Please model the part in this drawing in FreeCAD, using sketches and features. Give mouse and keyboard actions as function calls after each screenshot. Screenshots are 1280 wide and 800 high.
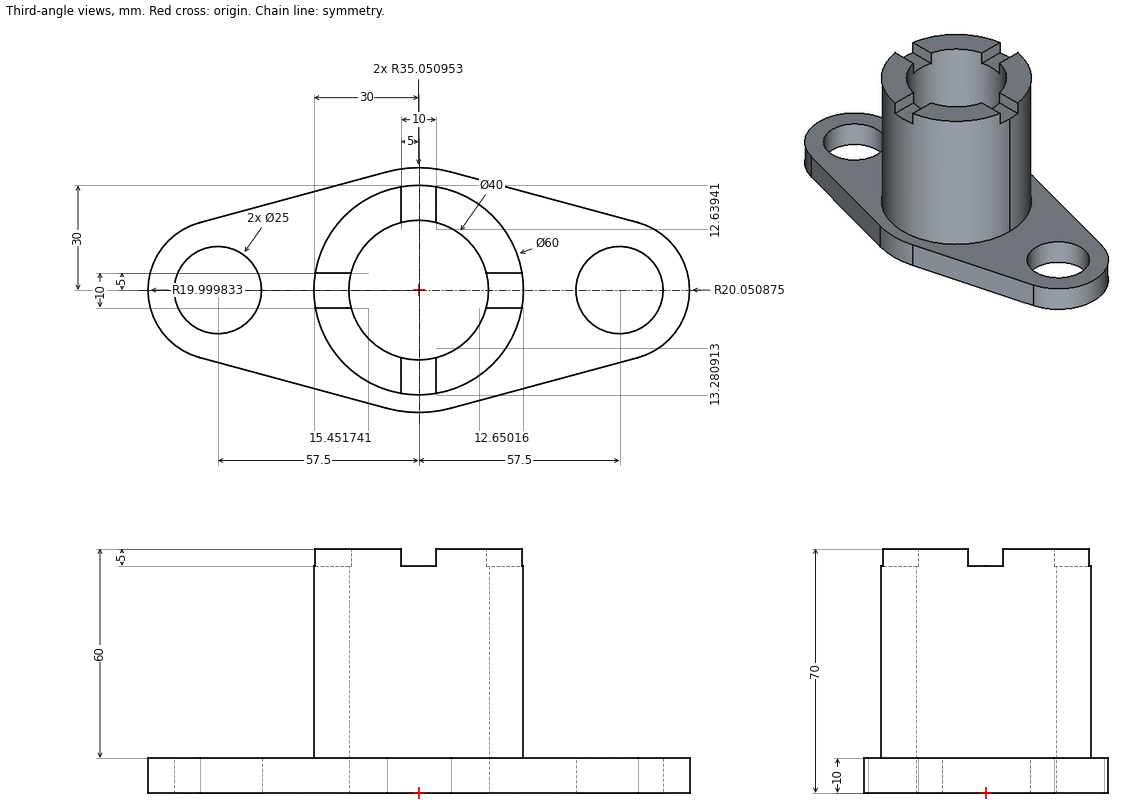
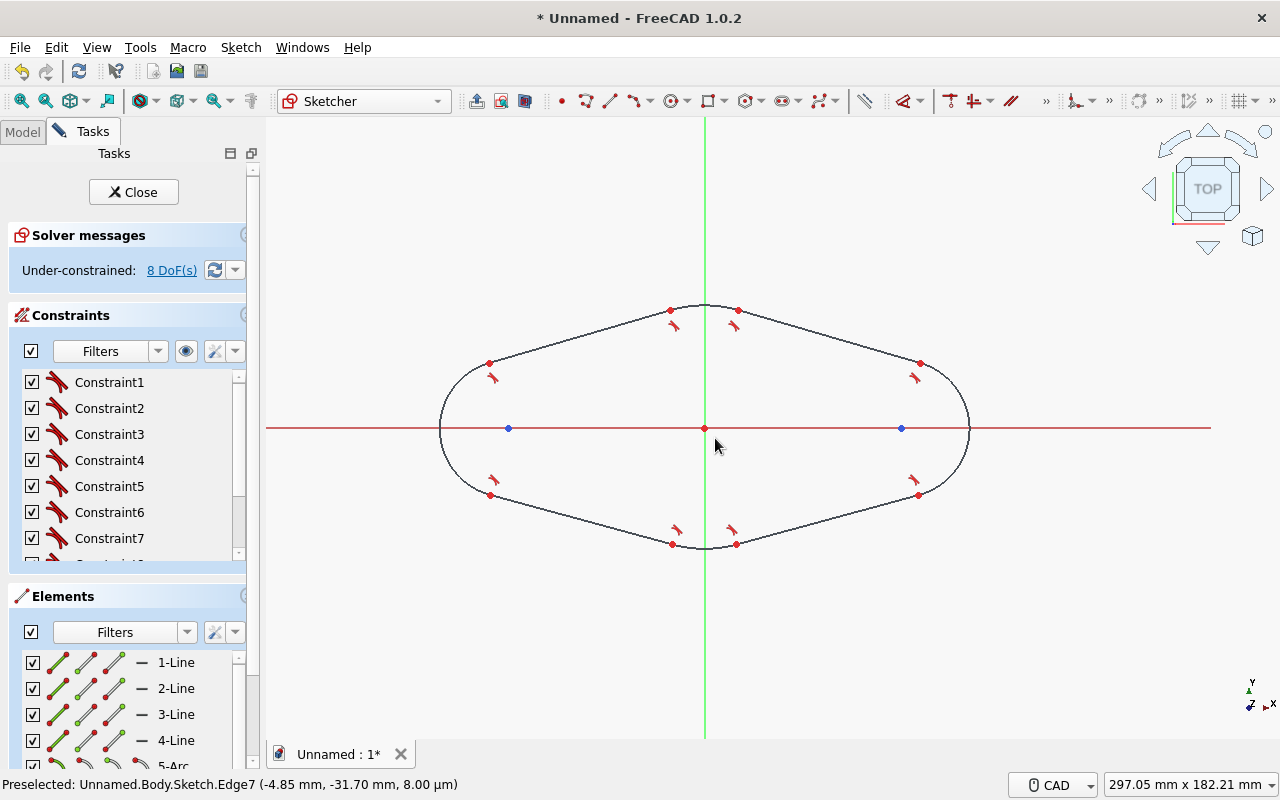
click(718, 306)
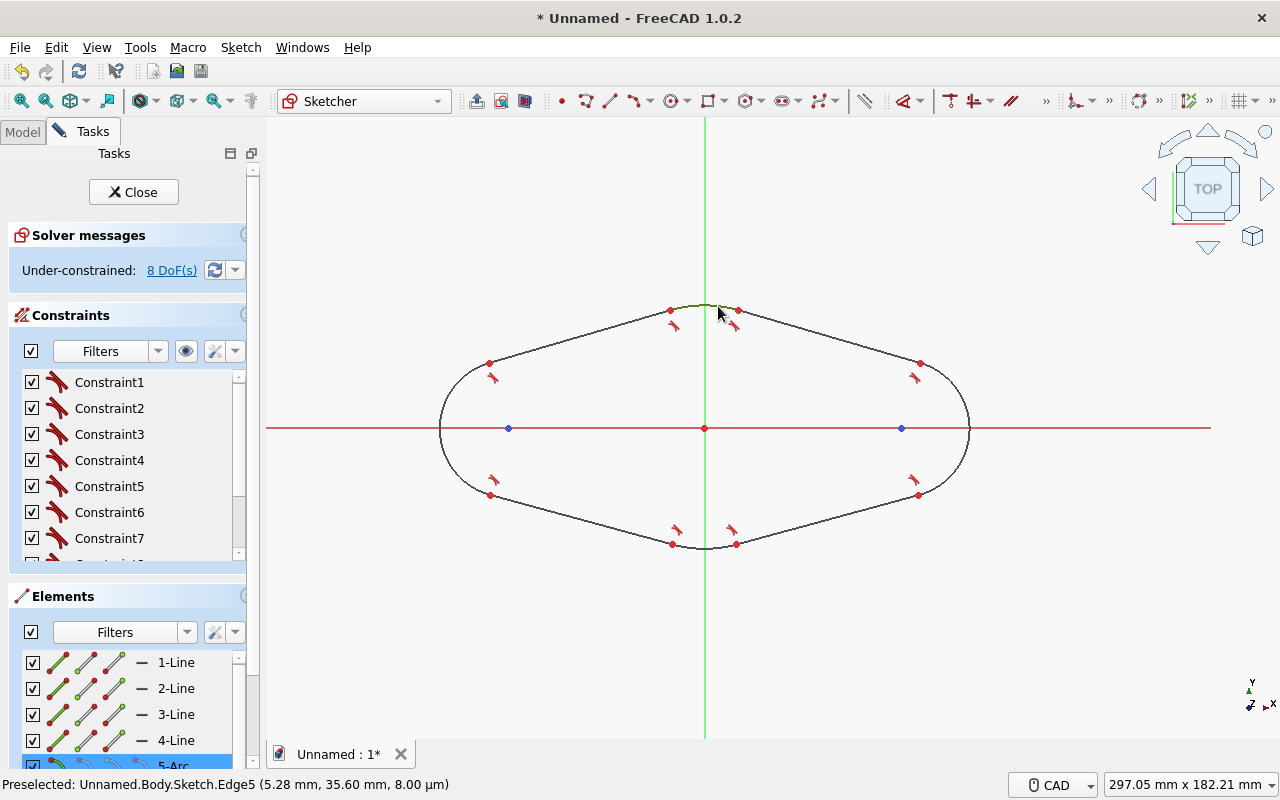
click(692, 548)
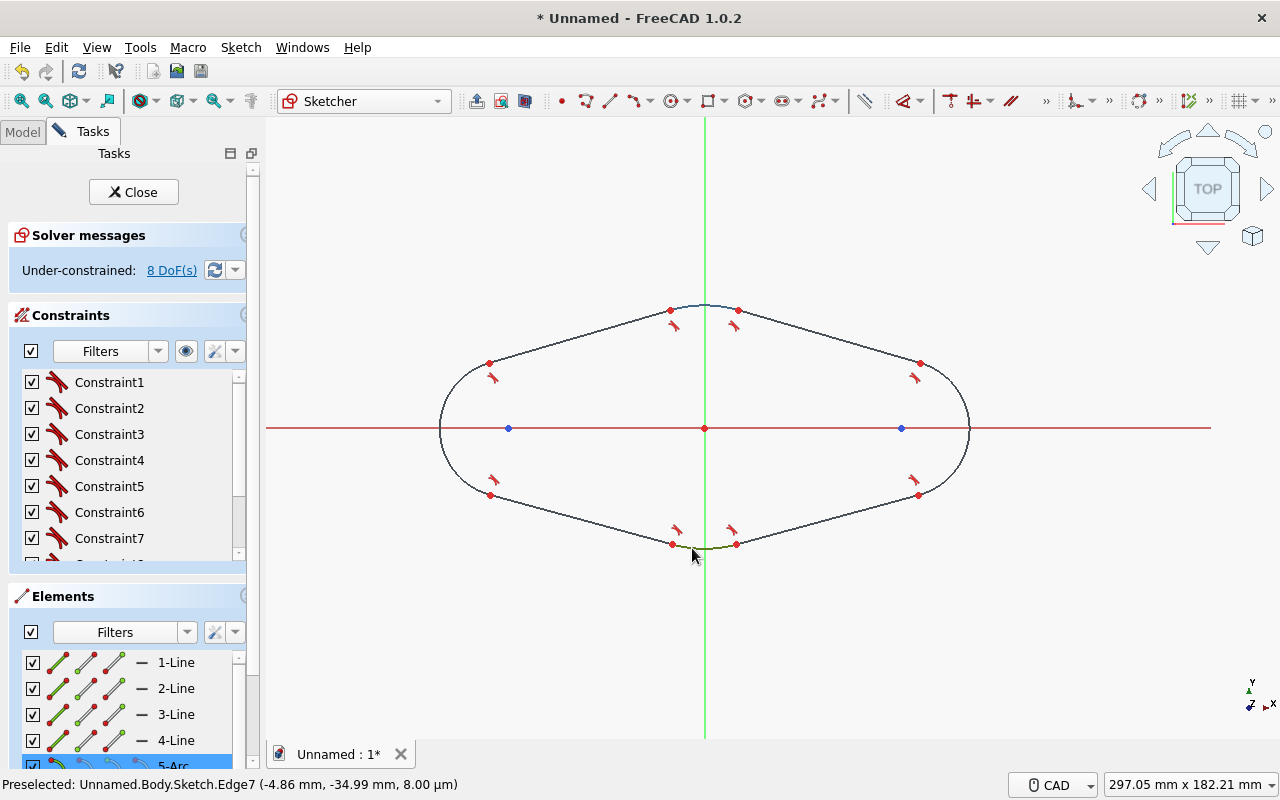
key(e)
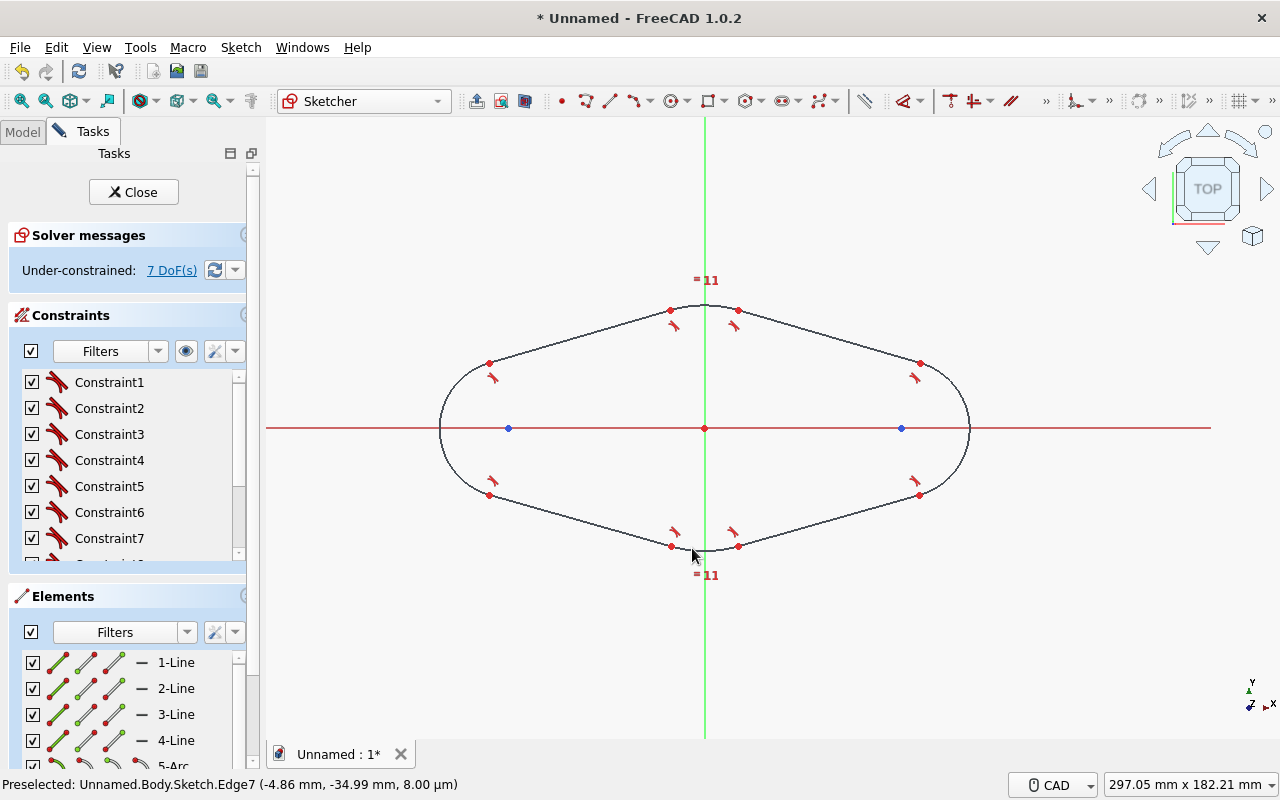
click(508, 429)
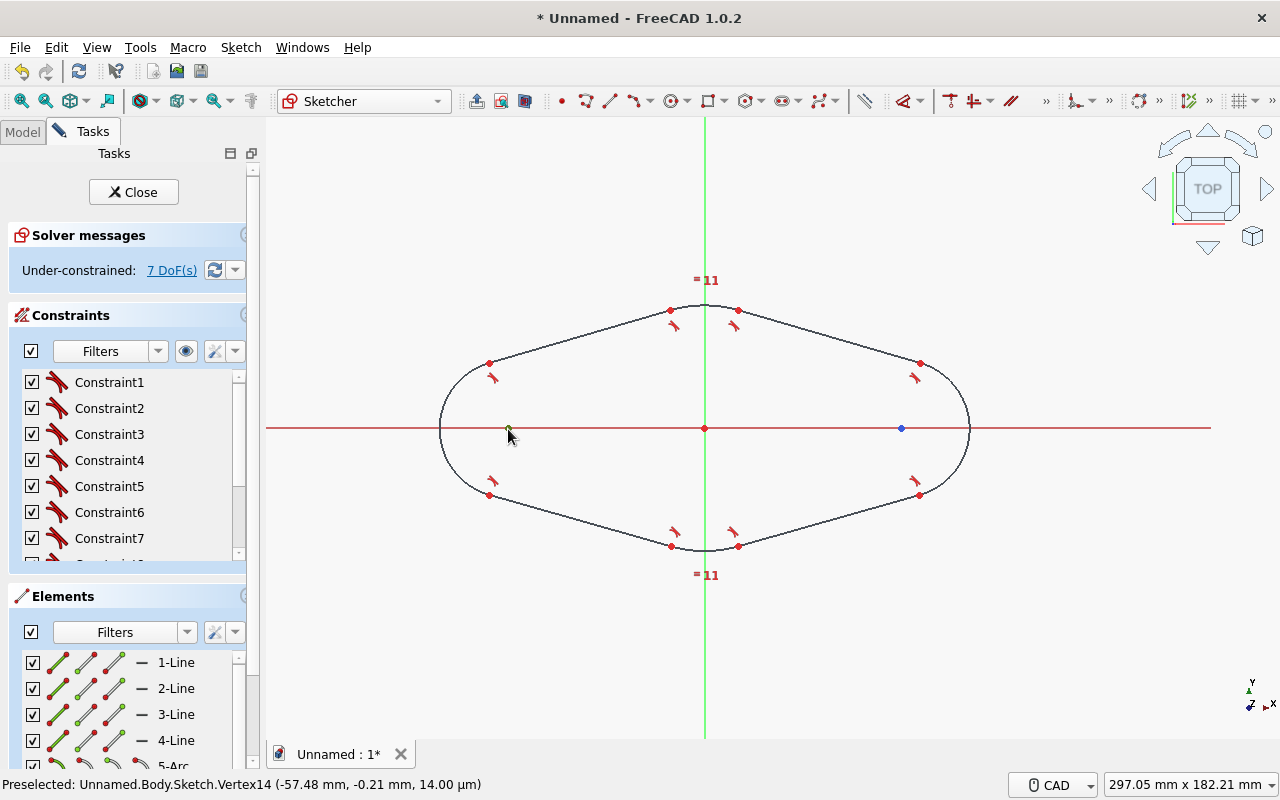
click(353, 428)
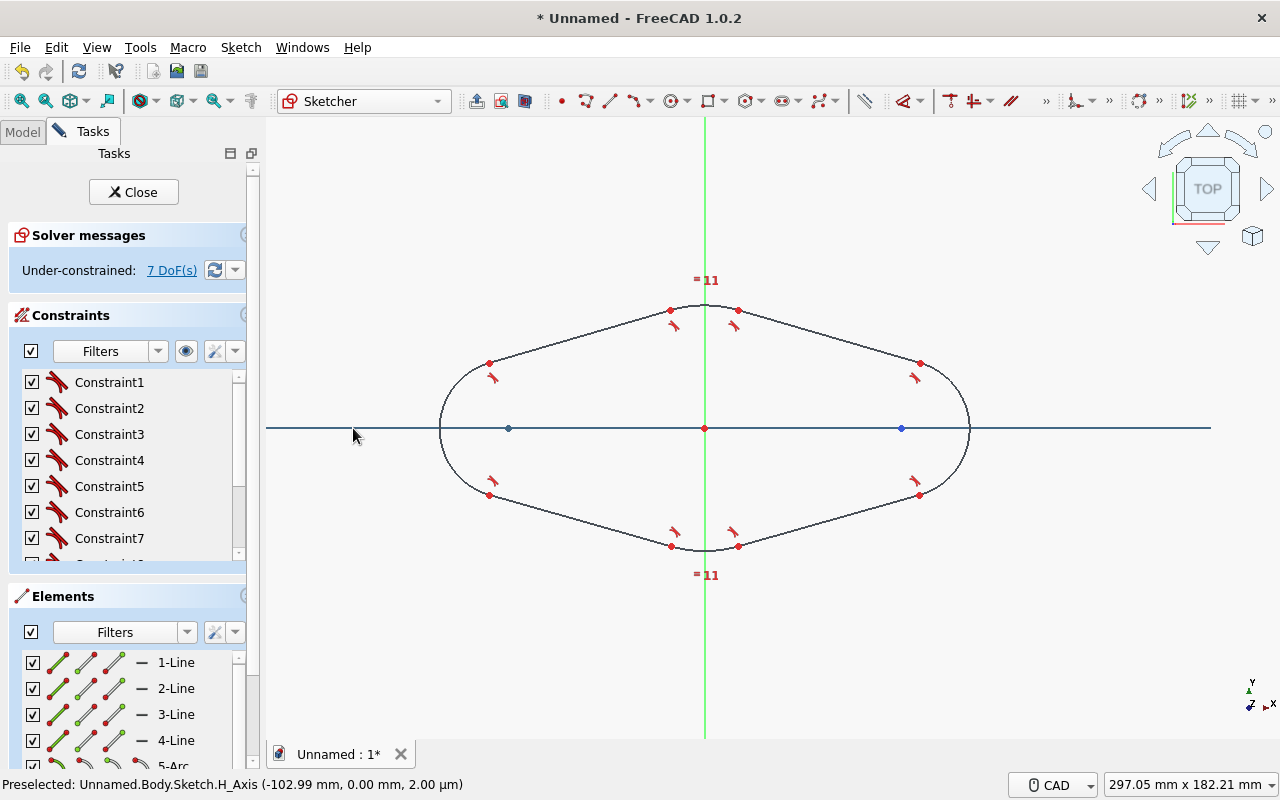
key(c)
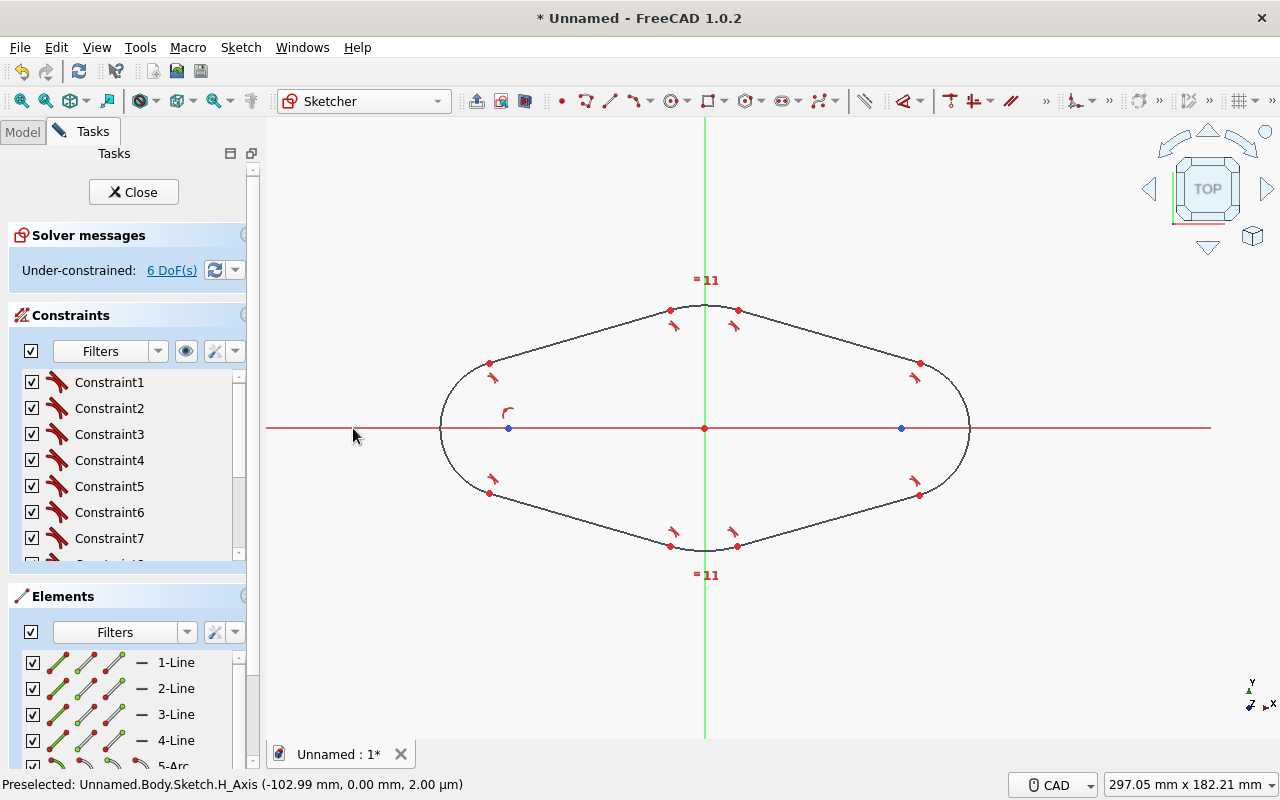
click(901, 429)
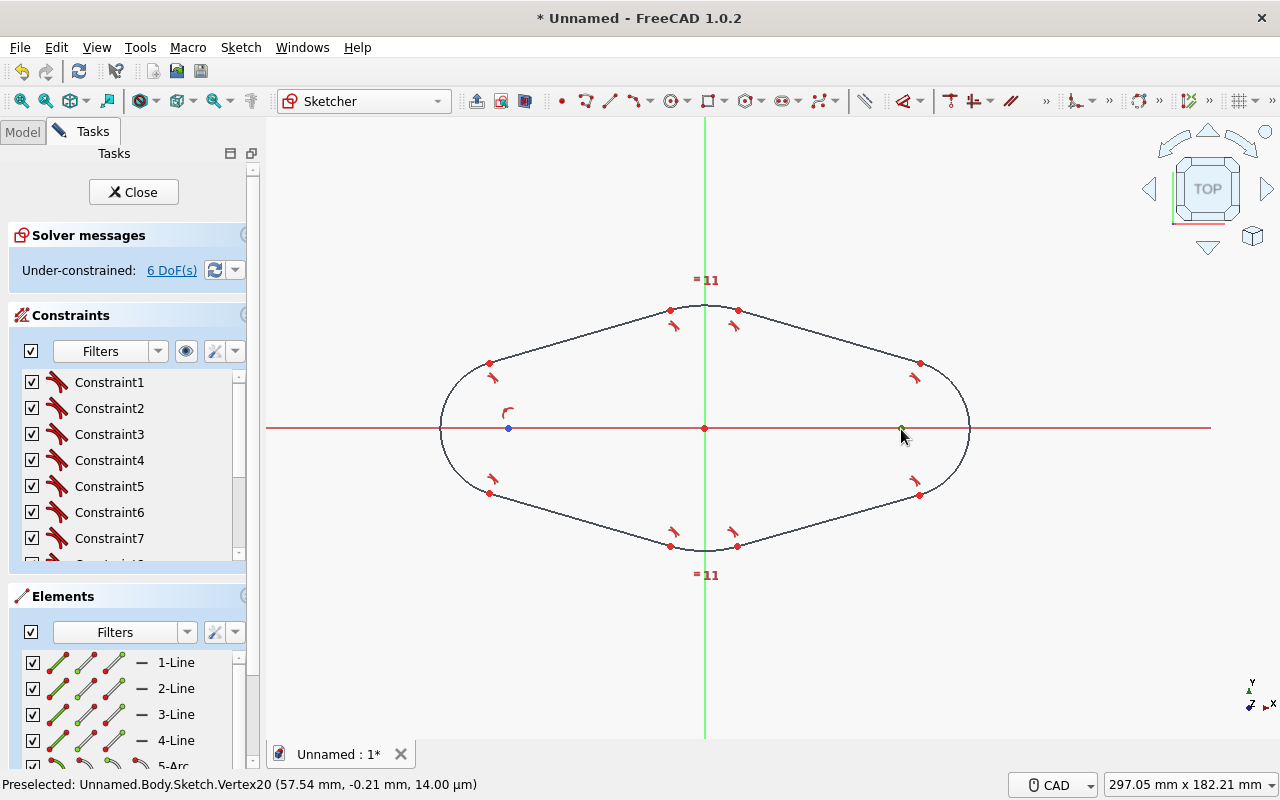
click(353, 428)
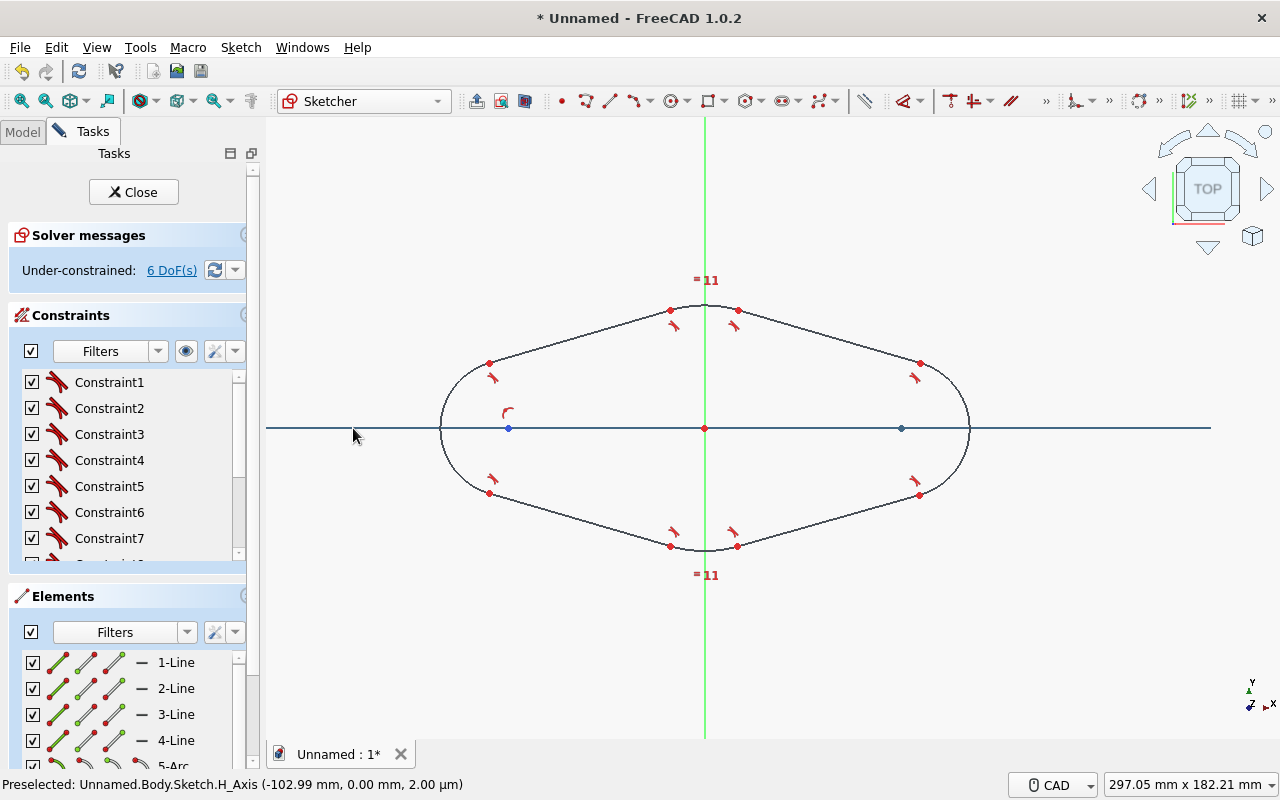
key(c)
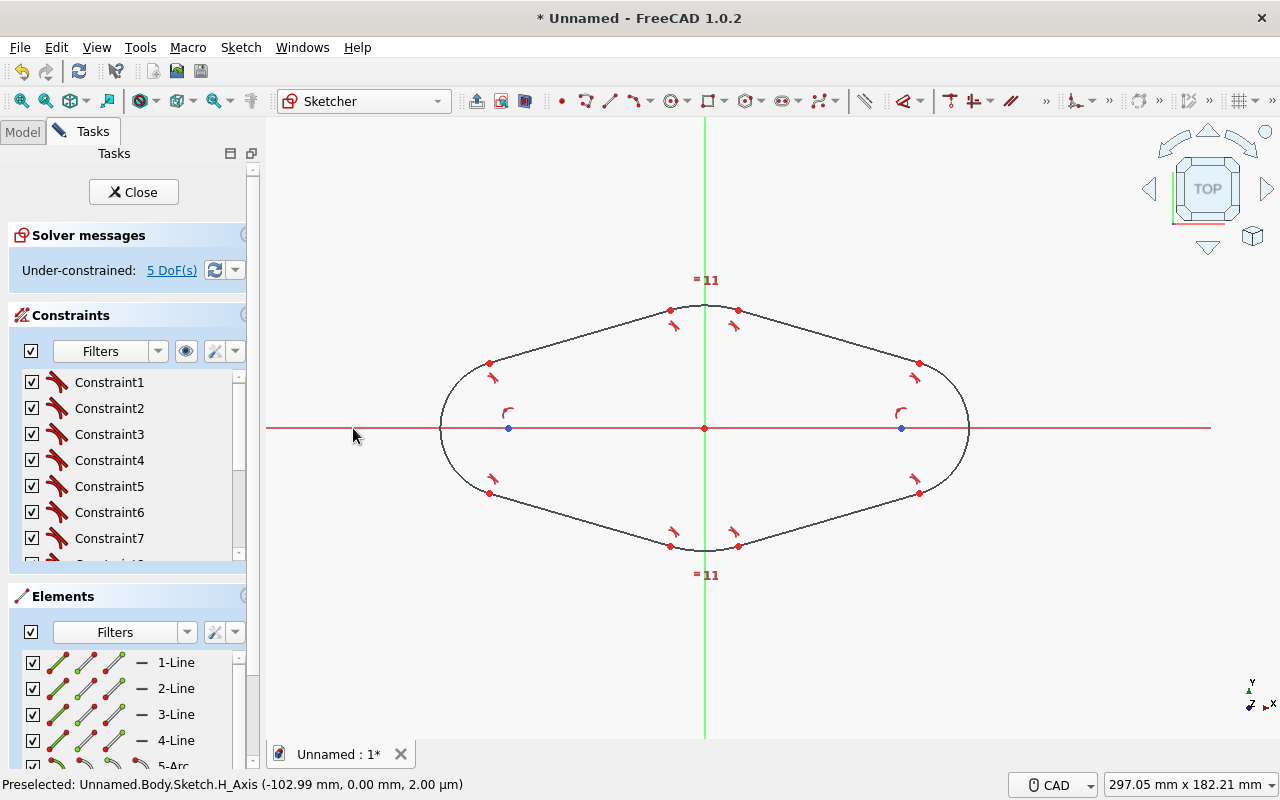
click(718, 306)